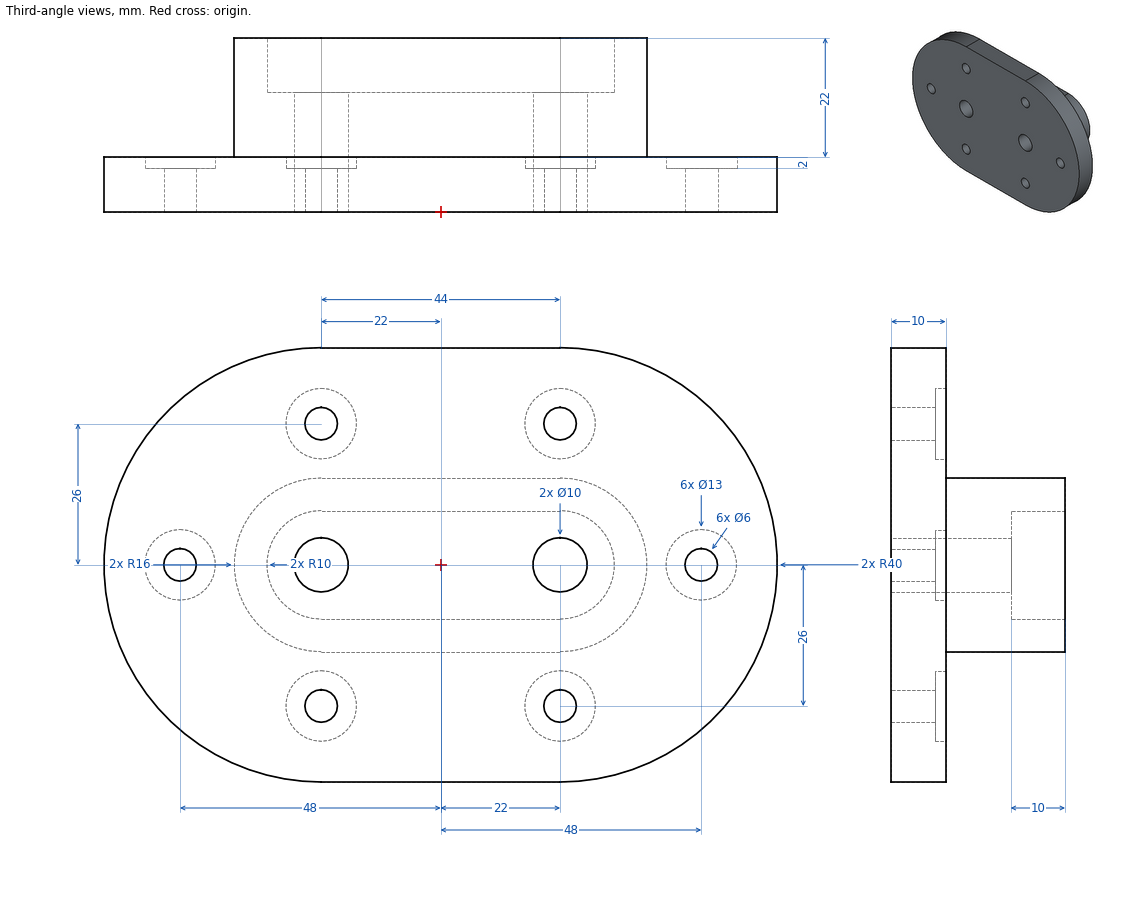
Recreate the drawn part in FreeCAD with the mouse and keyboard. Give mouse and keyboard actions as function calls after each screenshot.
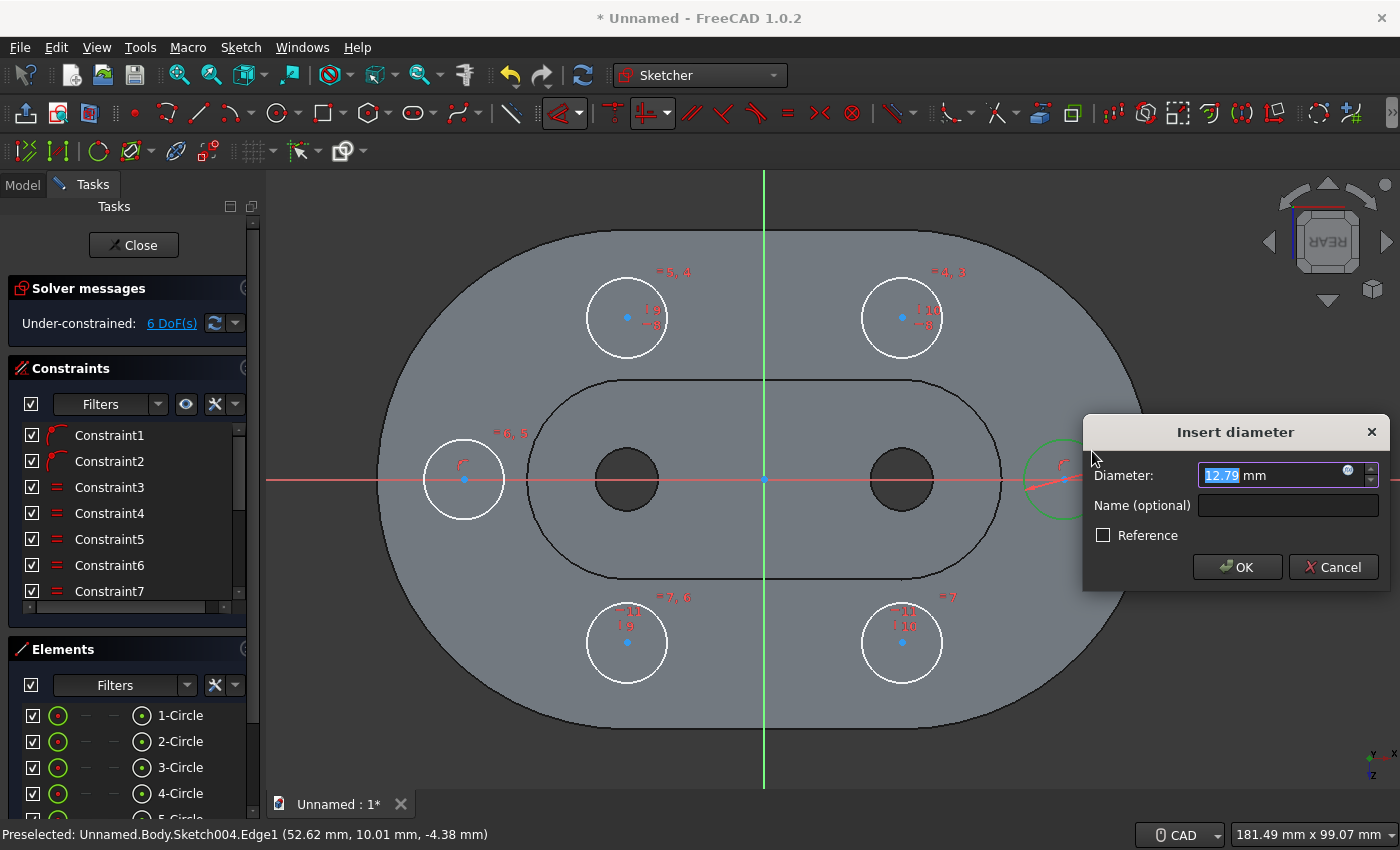
text(13)
key(Return)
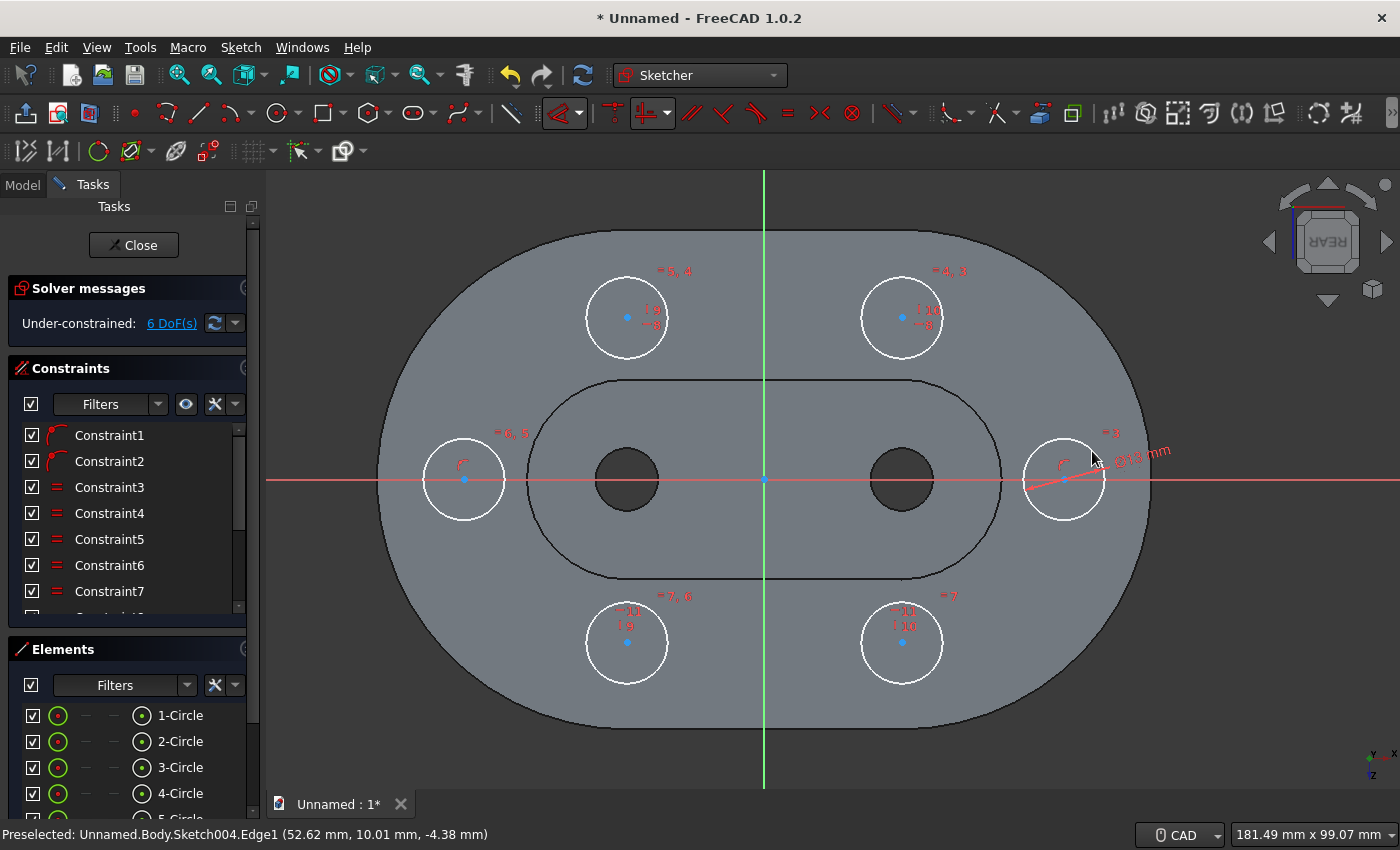
click(1064, 479)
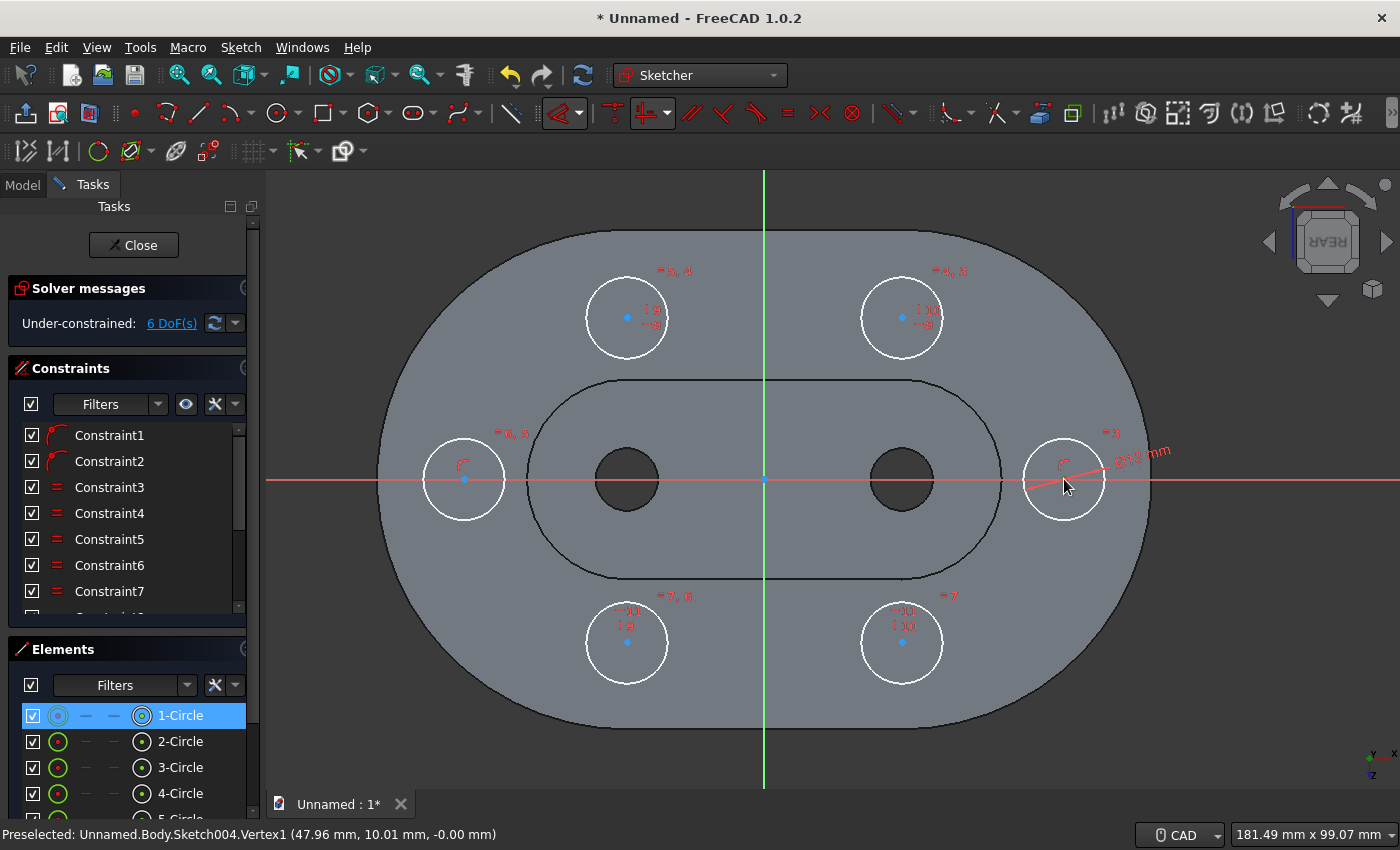
click(582, 114)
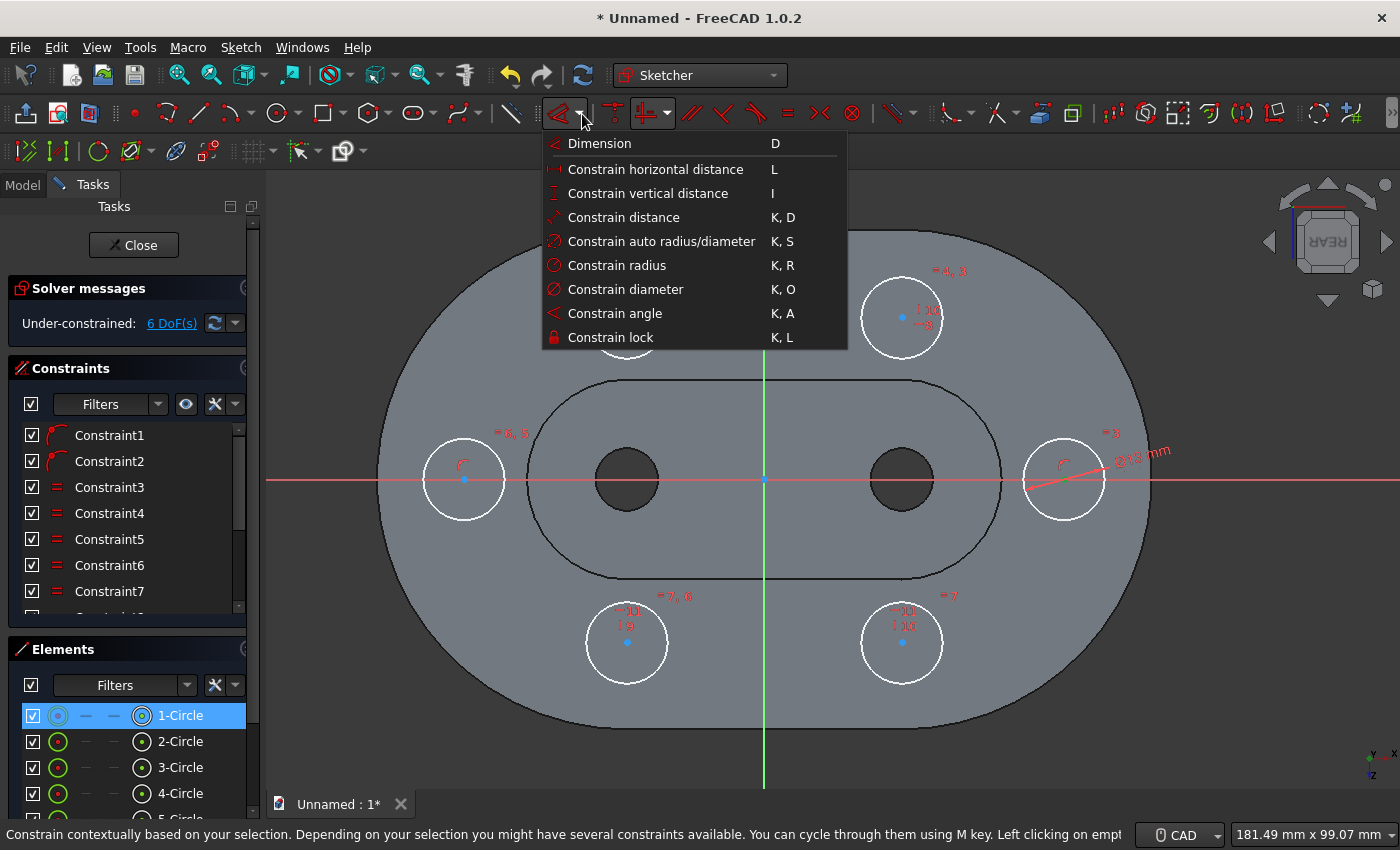
click(695, 169)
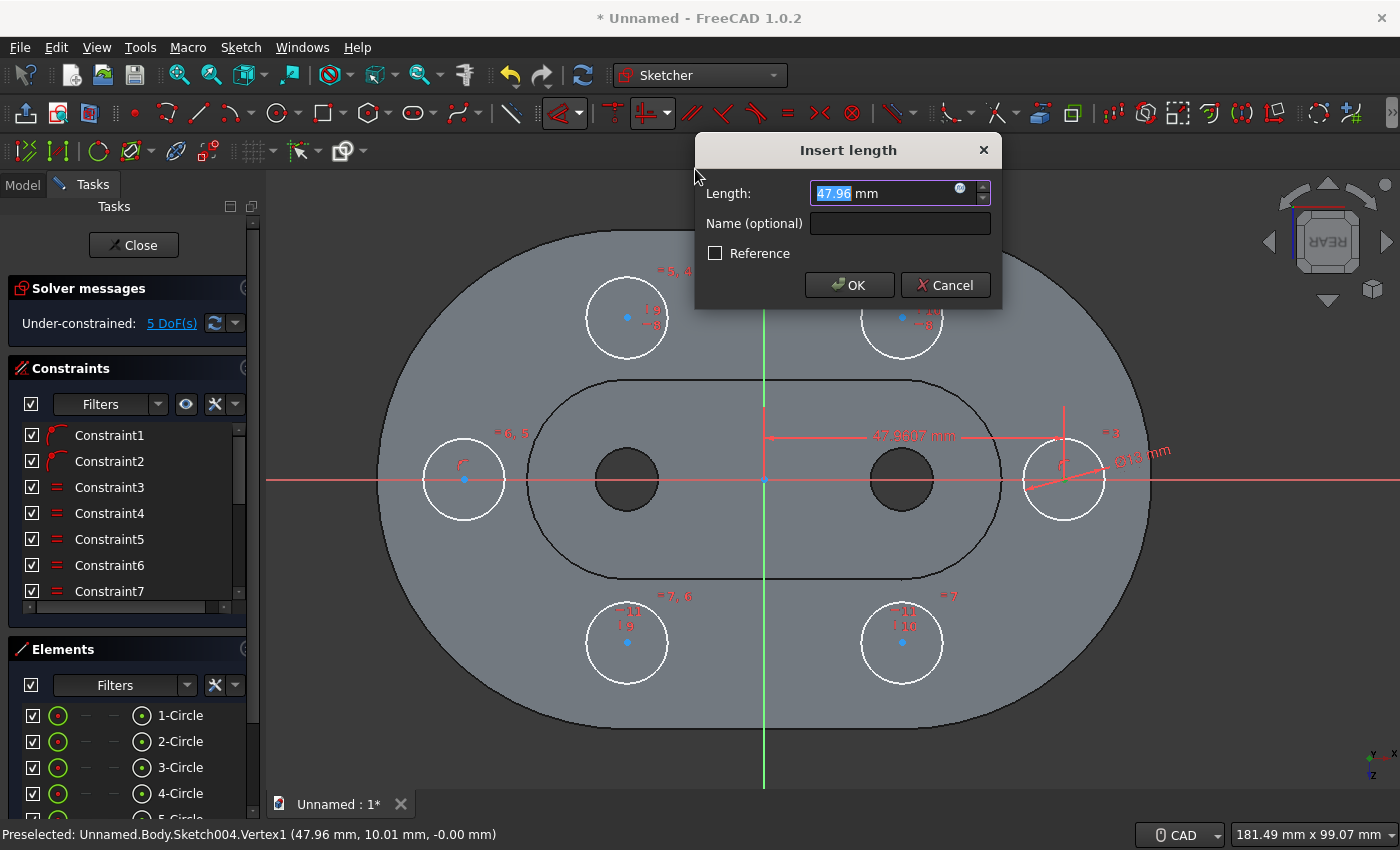
text(48)
key(Return)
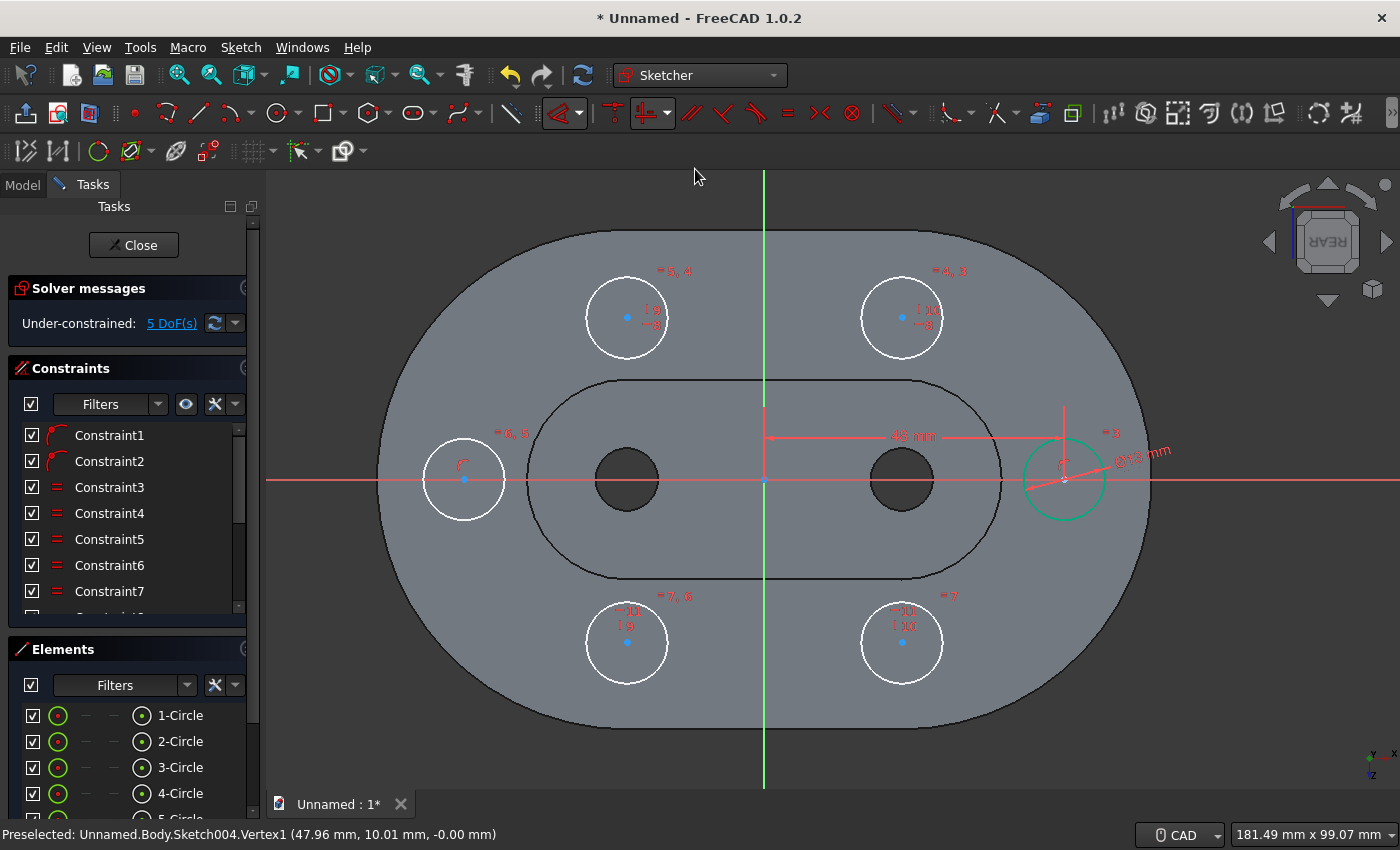
click(902, 318)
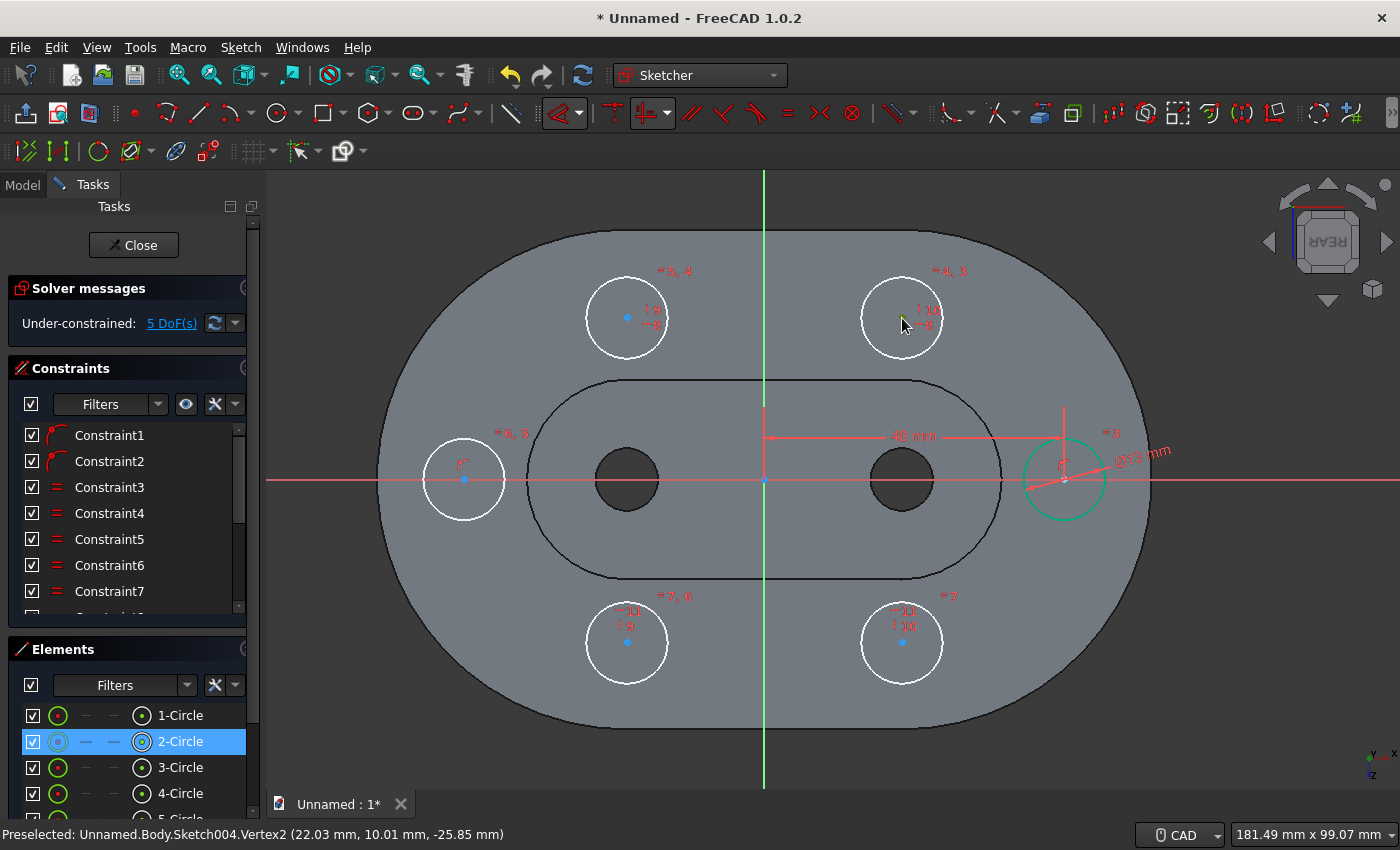
click(582, 114)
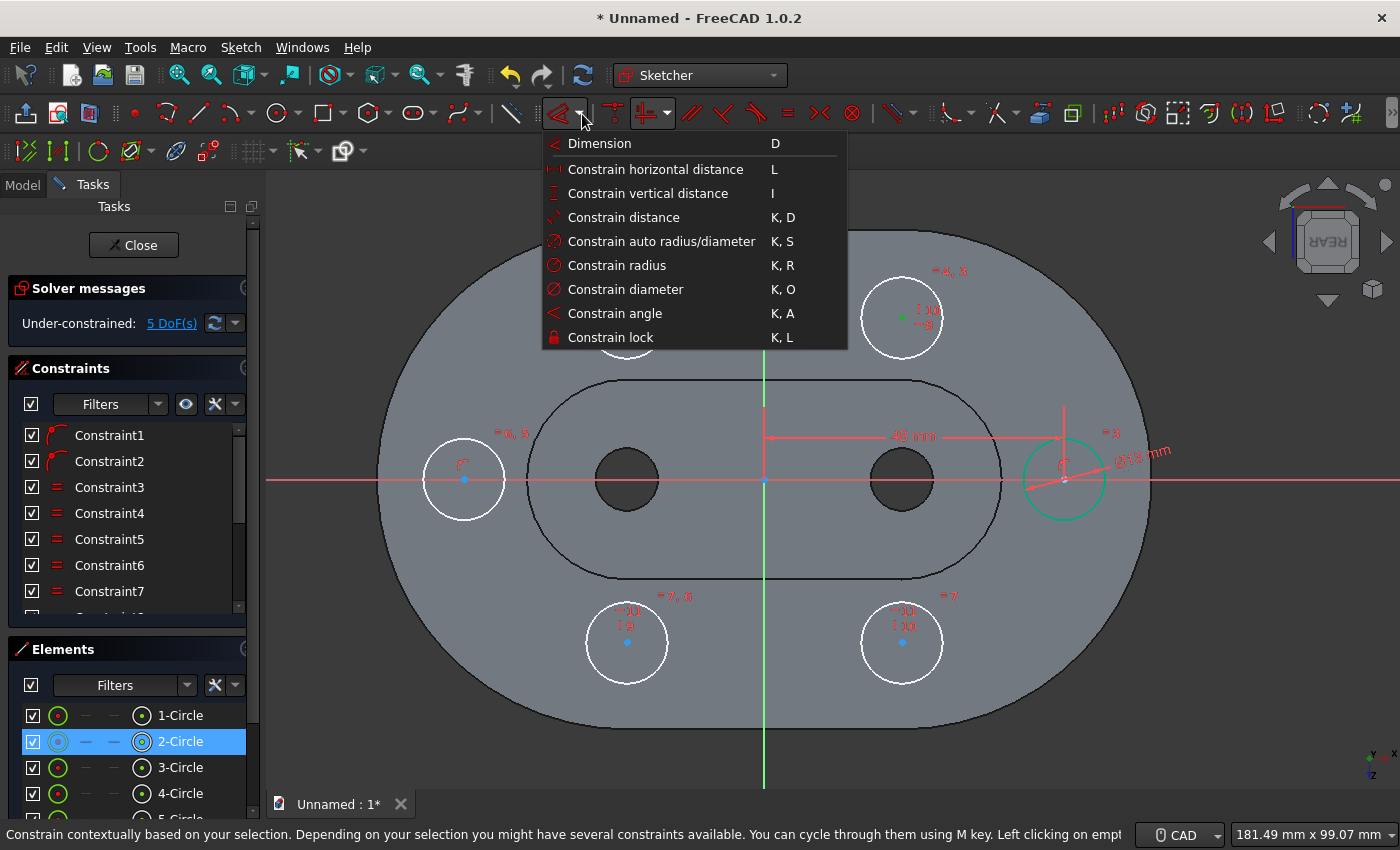
click(695, 169)